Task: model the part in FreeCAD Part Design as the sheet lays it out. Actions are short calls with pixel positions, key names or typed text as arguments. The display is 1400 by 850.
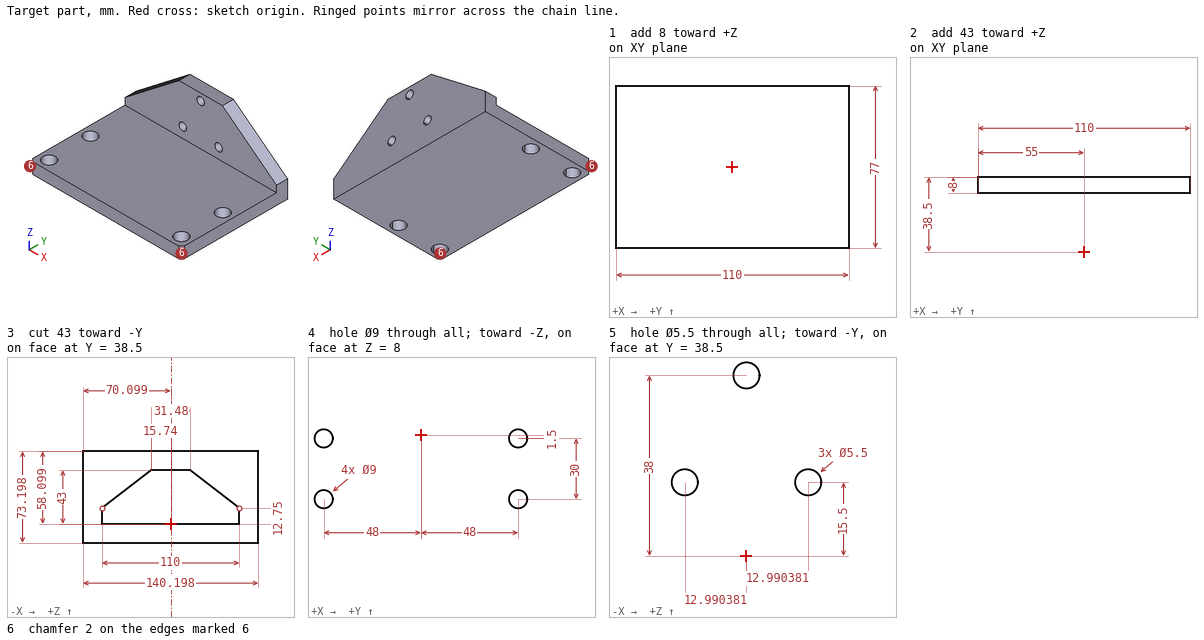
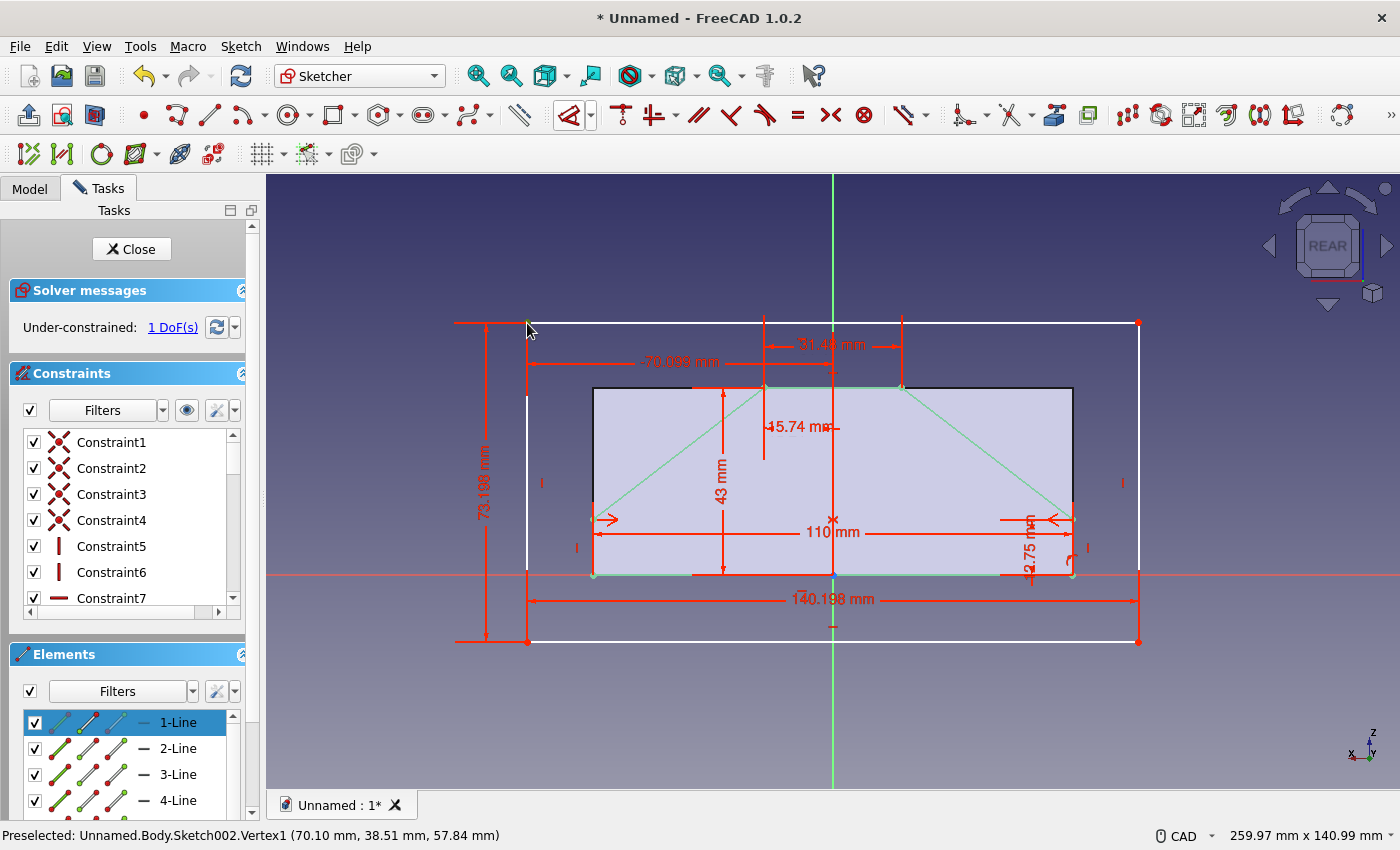
key(i)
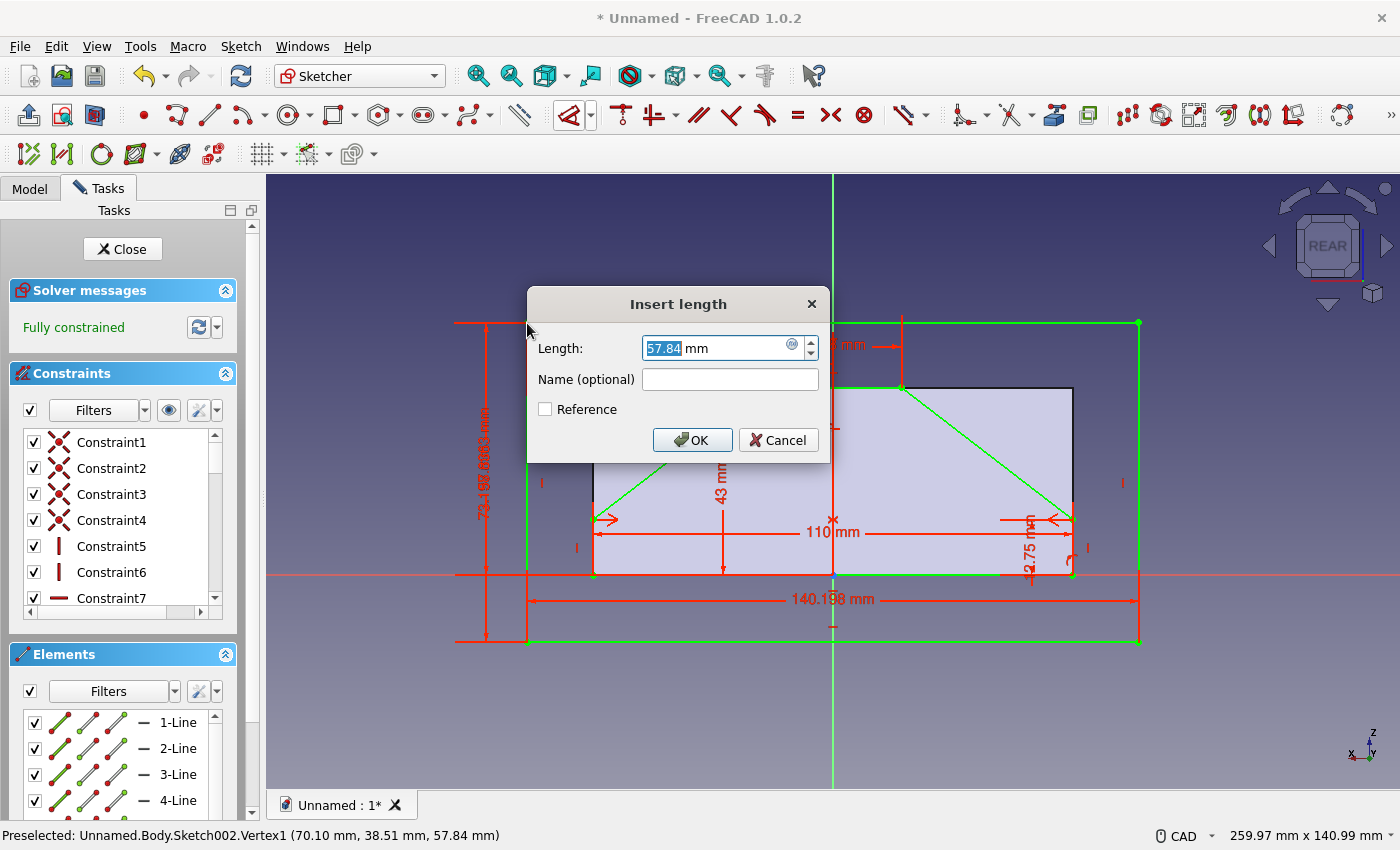
text(58.099)
key(Return)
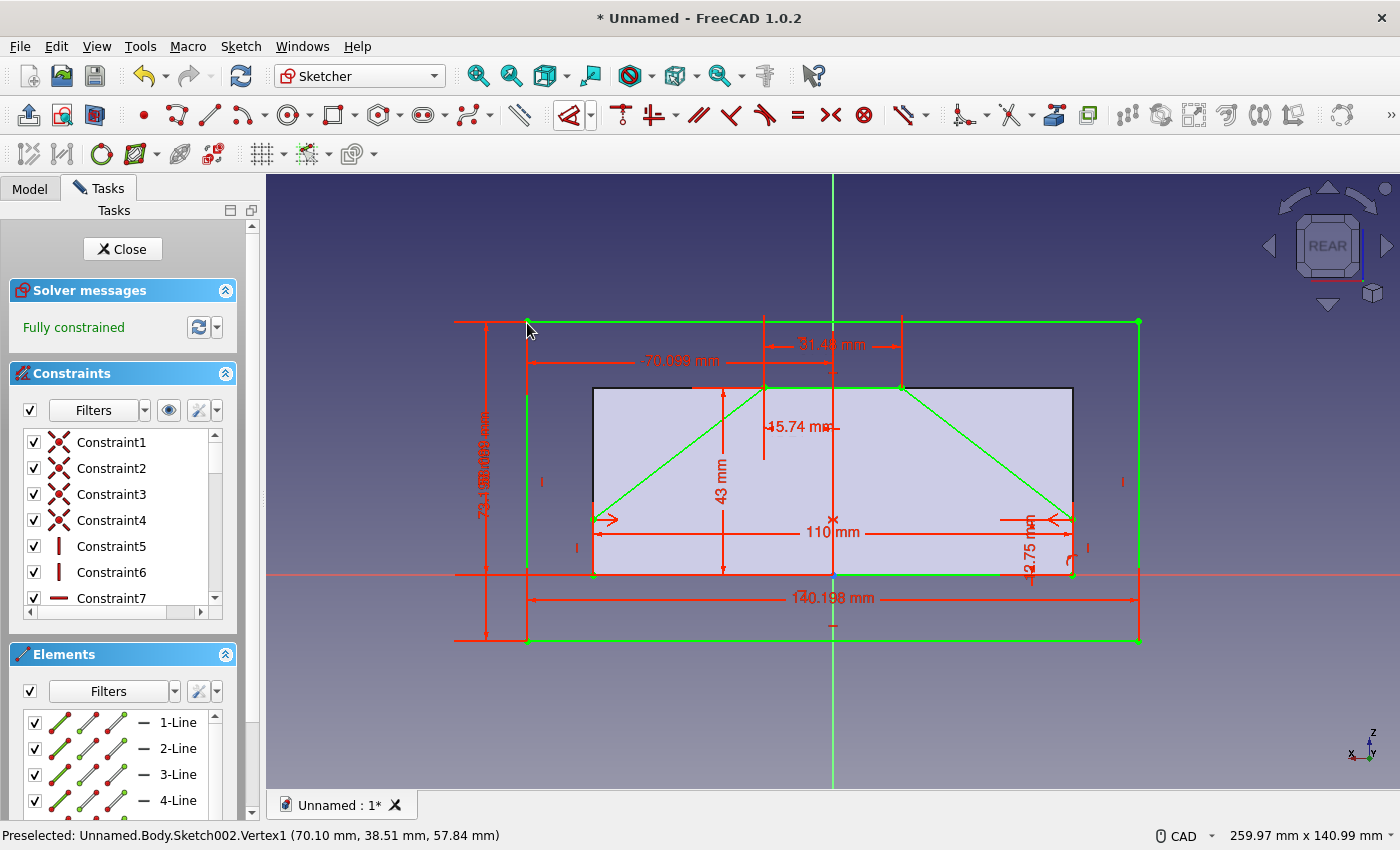
click(123, 249)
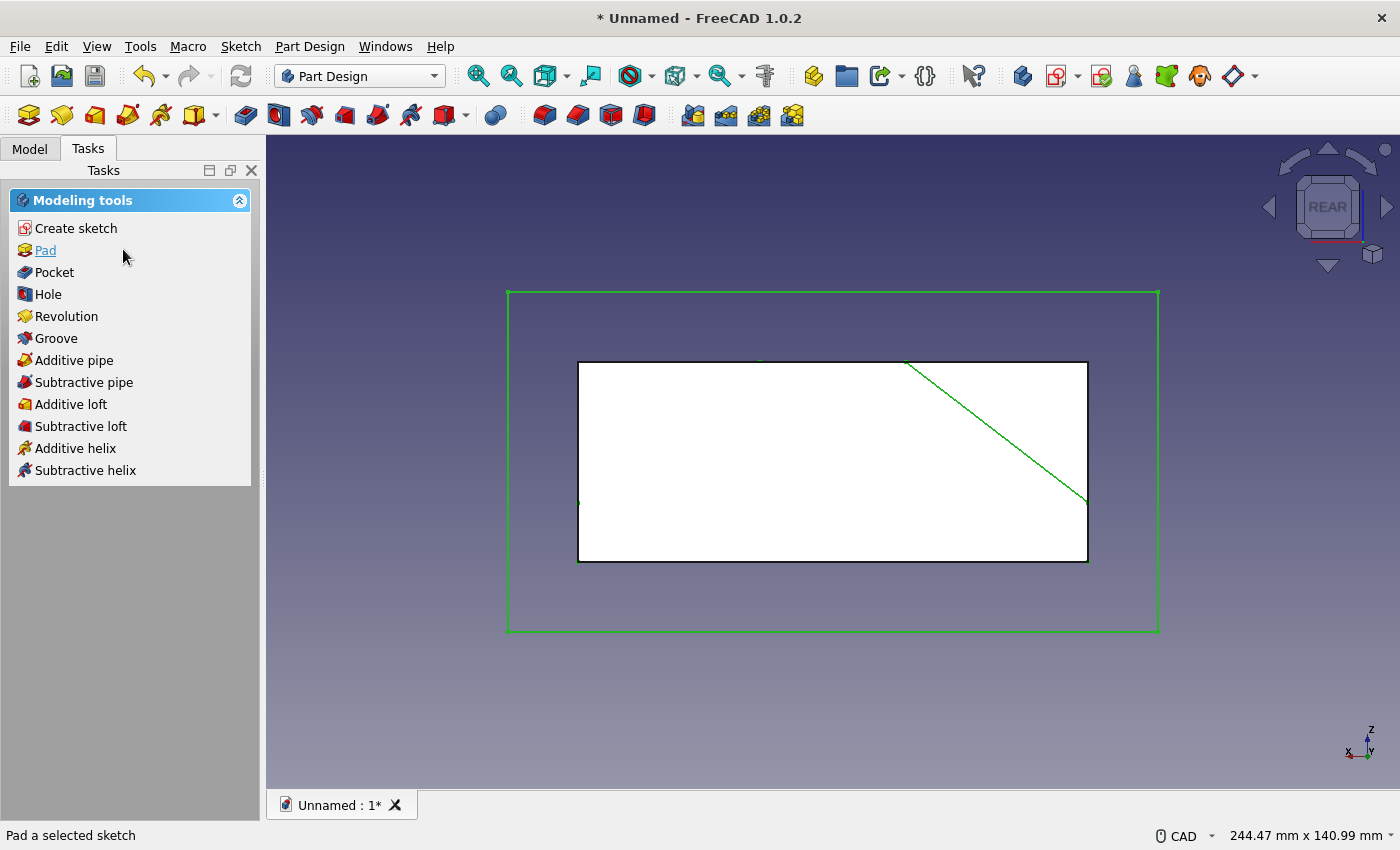
click(246, 116)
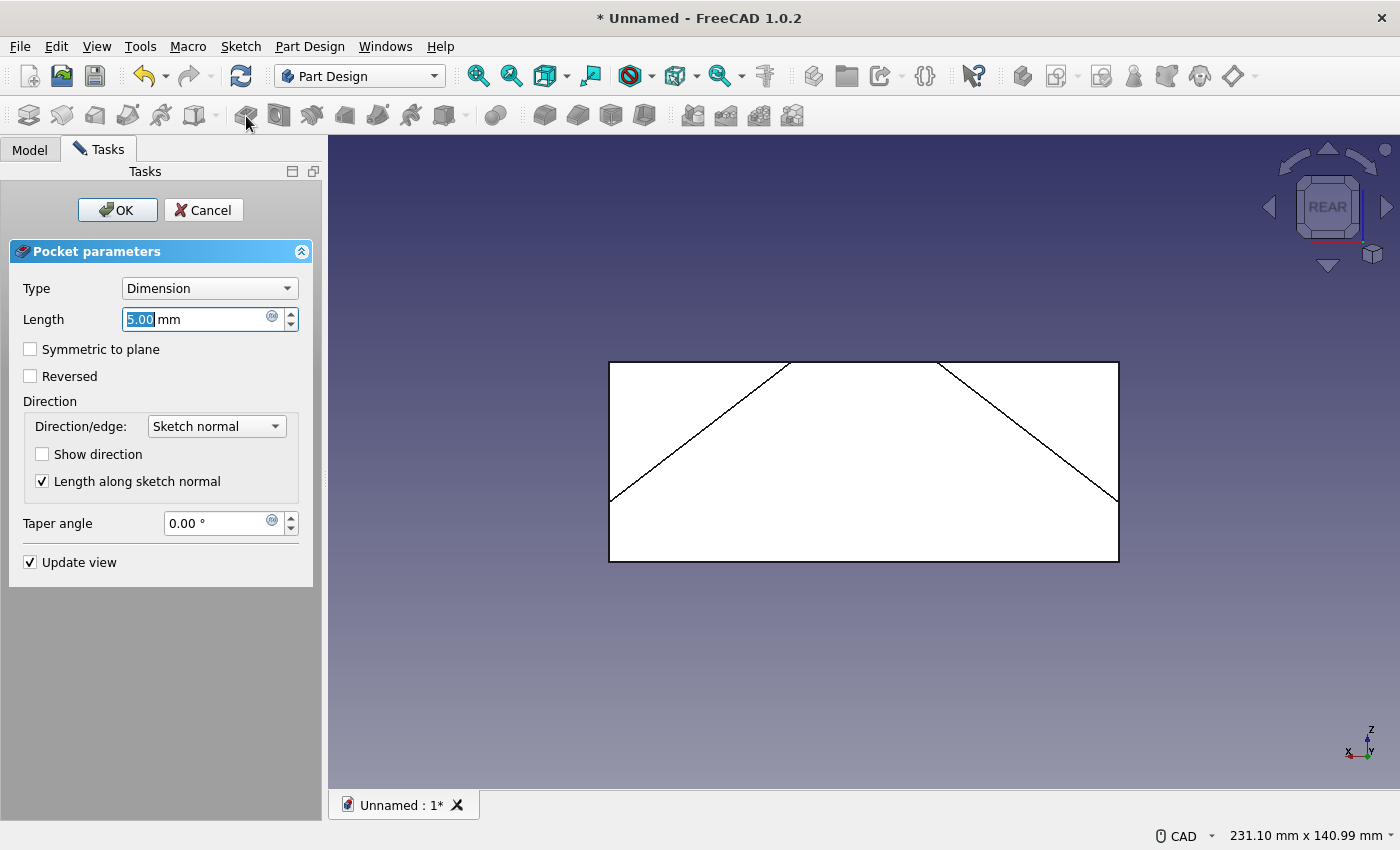
text(43)
key(Tab)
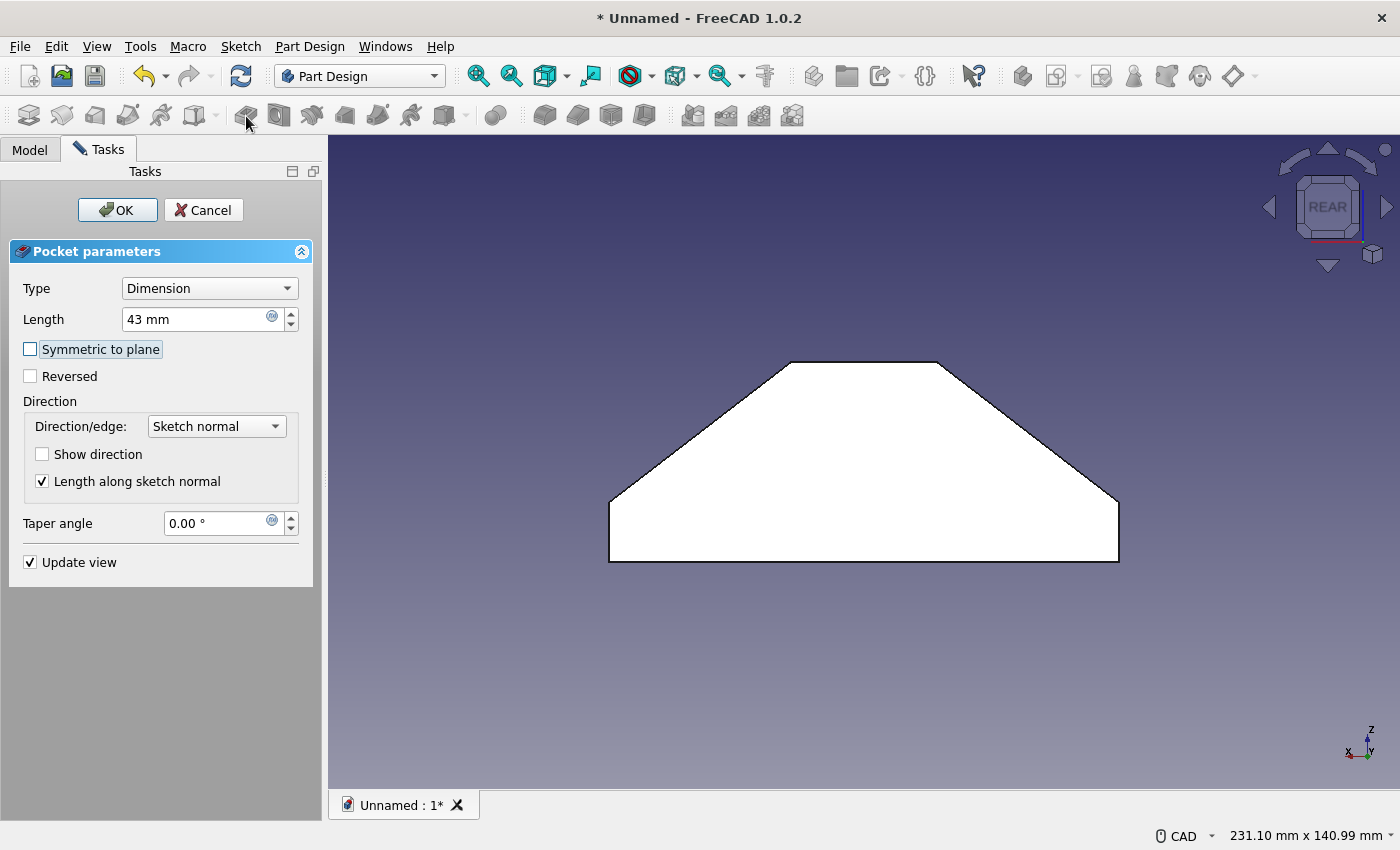
click(118, 210)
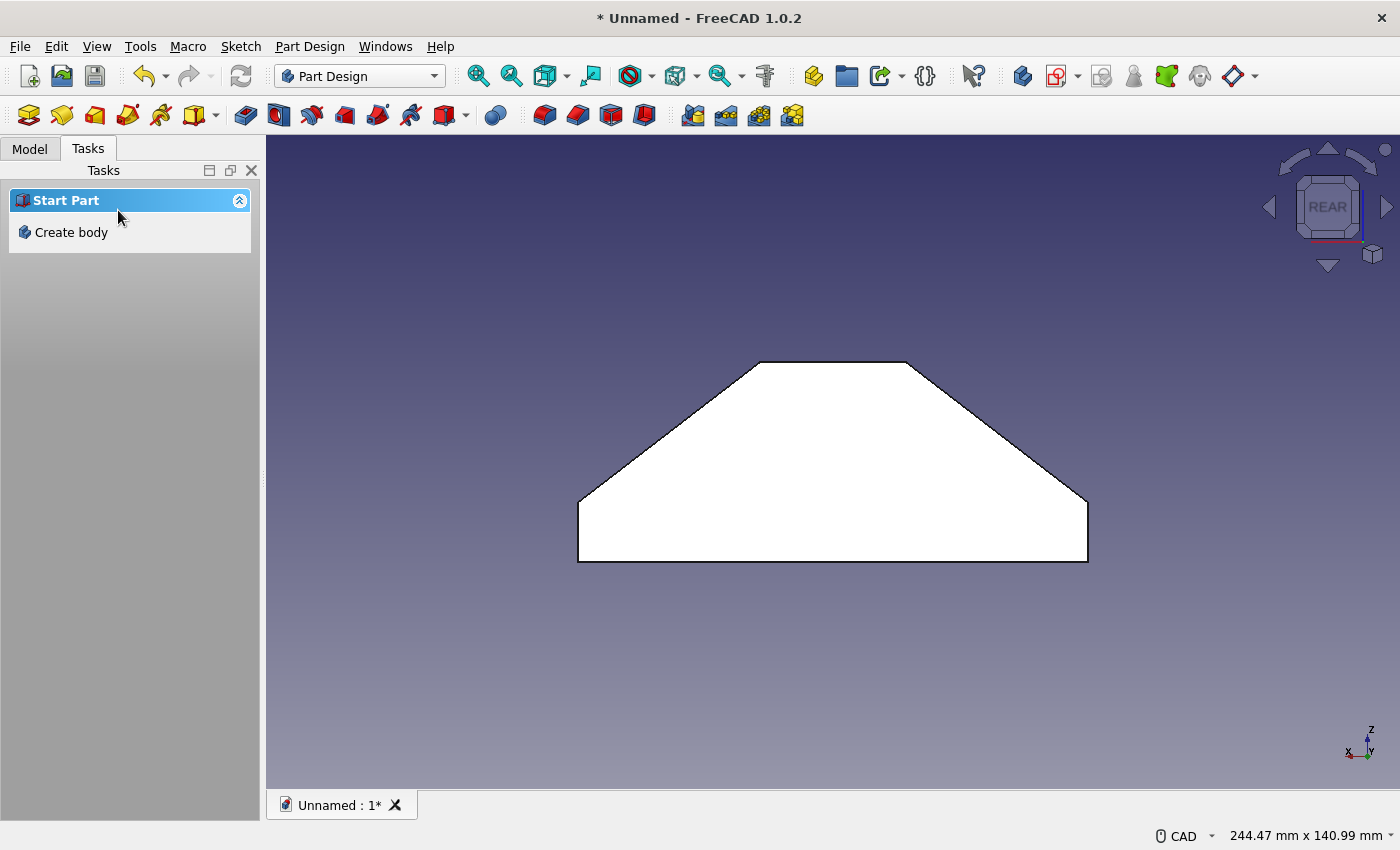
key(v)
key(f)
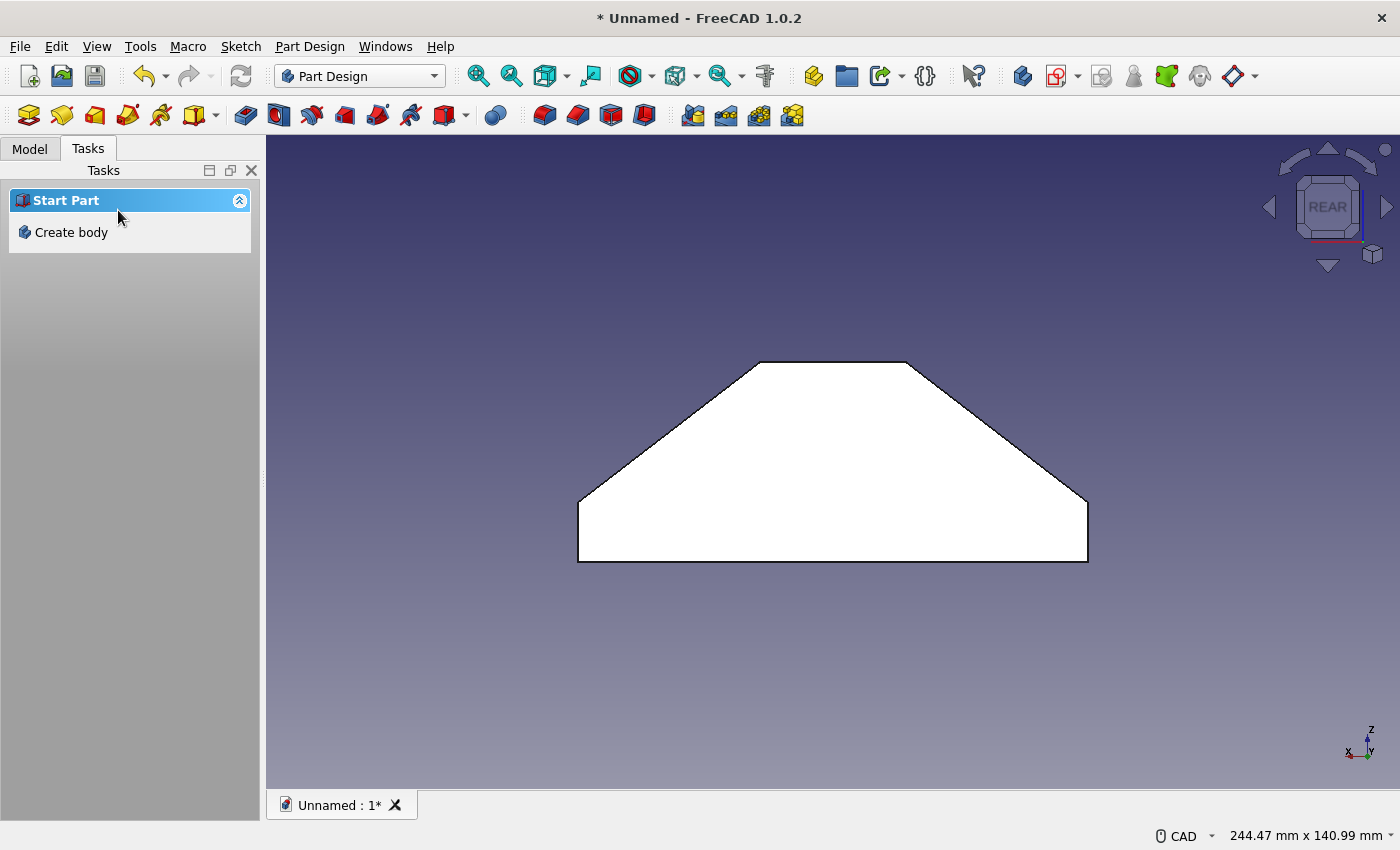
key(0)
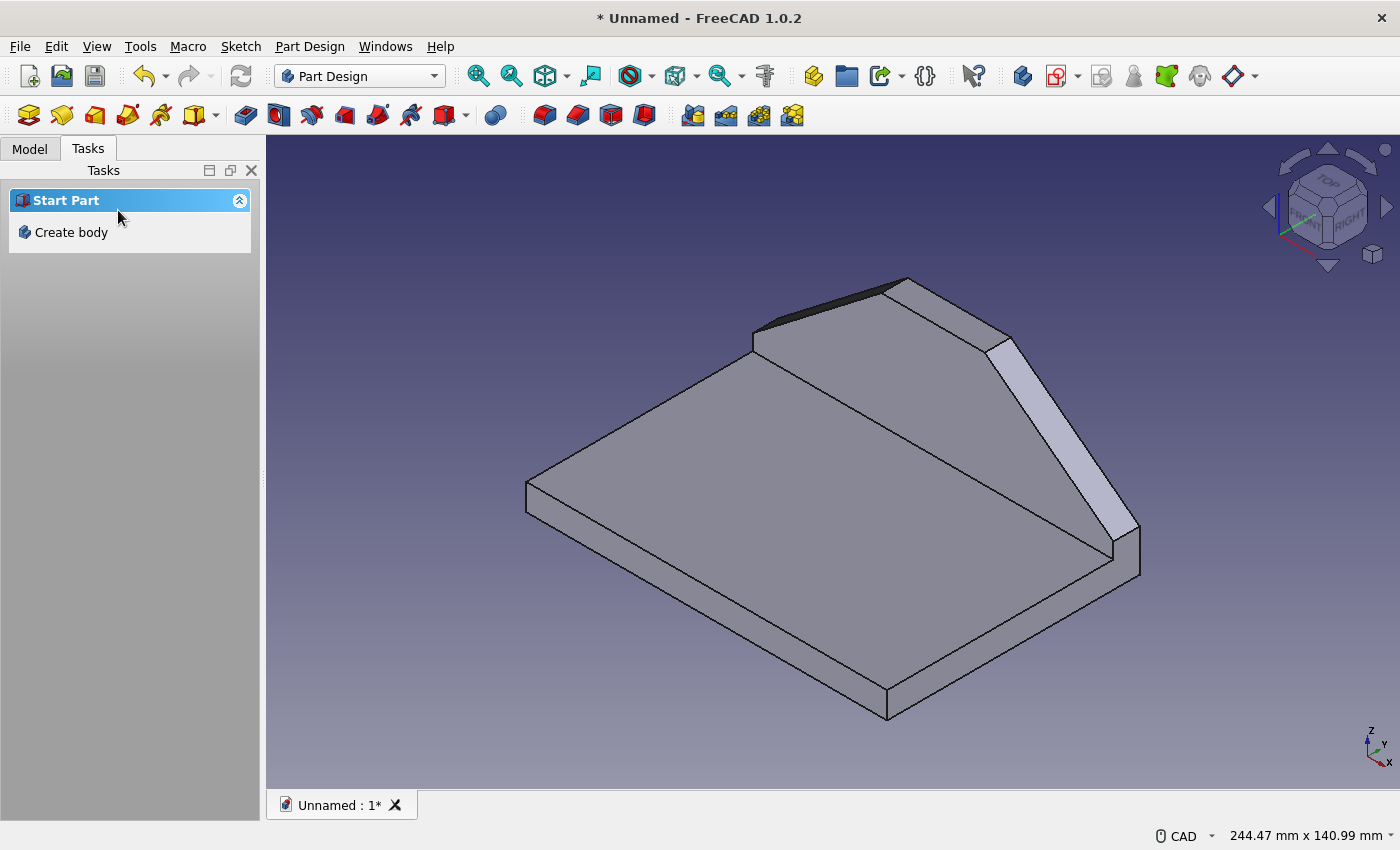
click(871, 549)